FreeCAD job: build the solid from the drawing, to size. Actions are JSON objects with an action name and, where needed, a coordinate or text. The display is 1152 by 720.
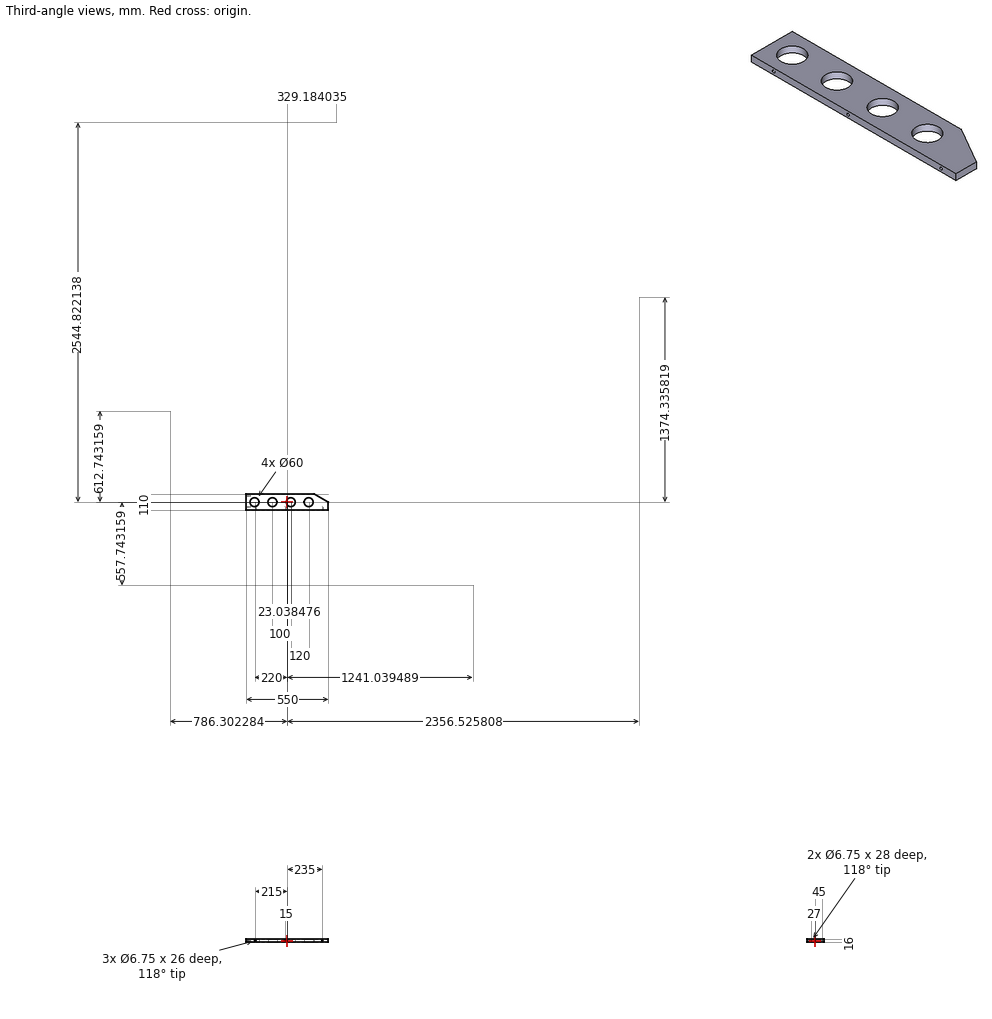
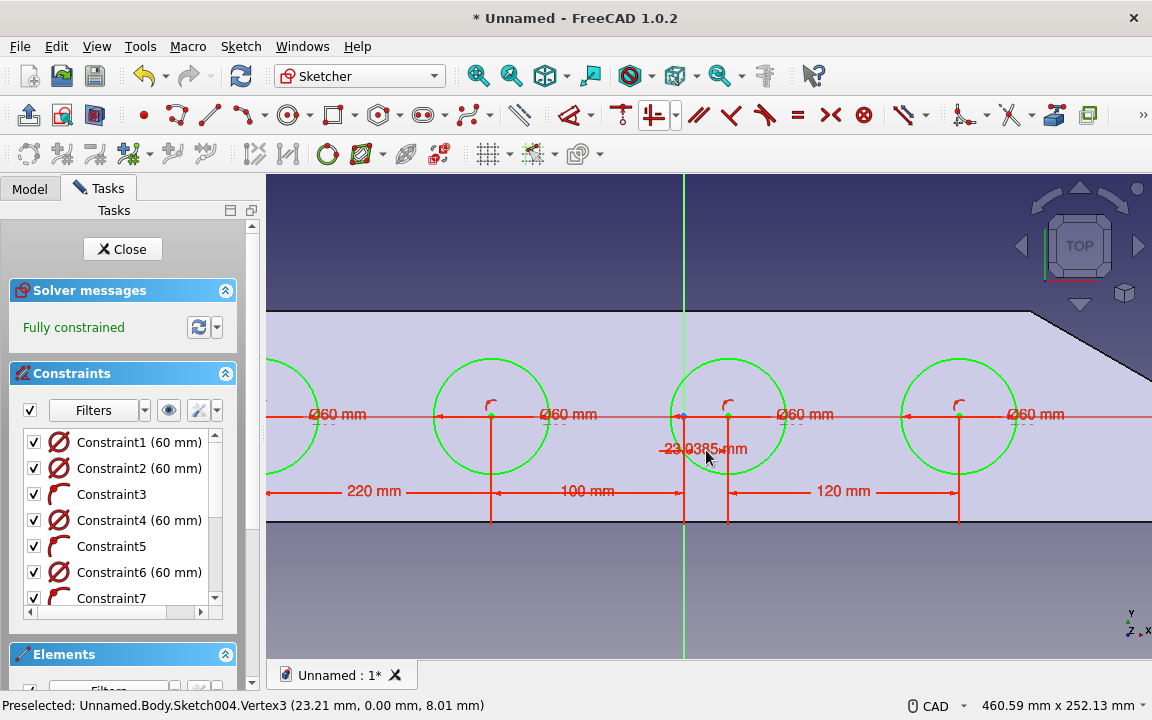
{"action": "left_click", "coordinate": [123, 249]}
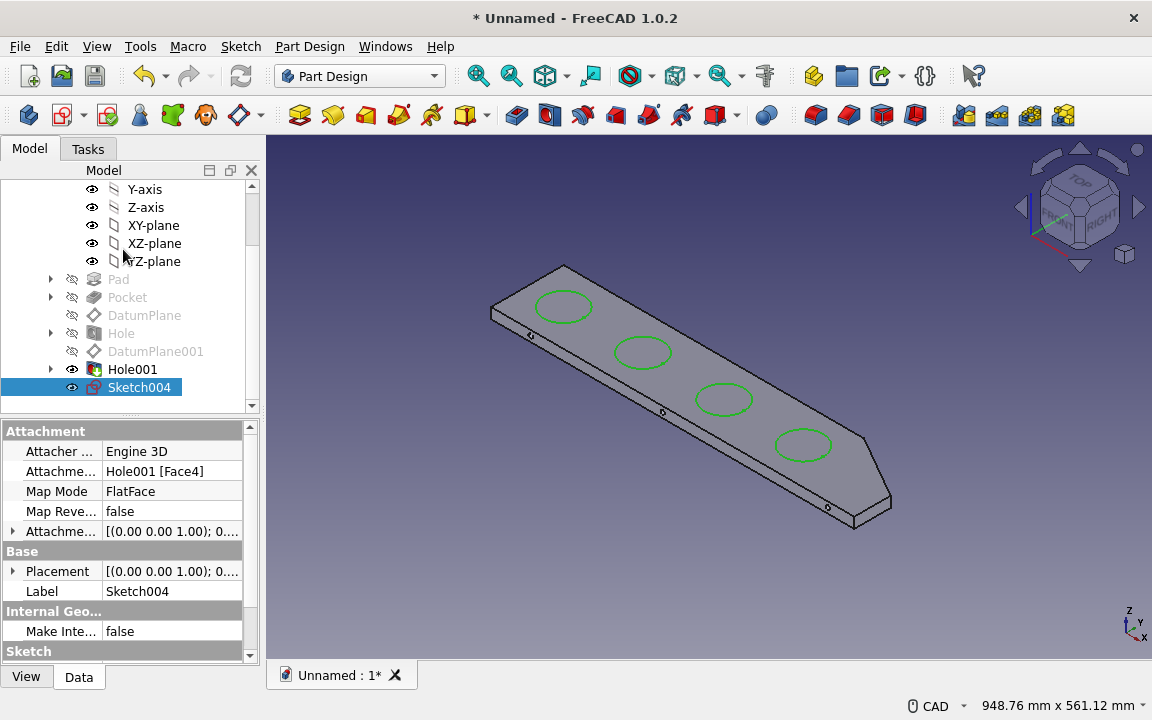
{"action": "left_click", "coordinate": [517, 116]}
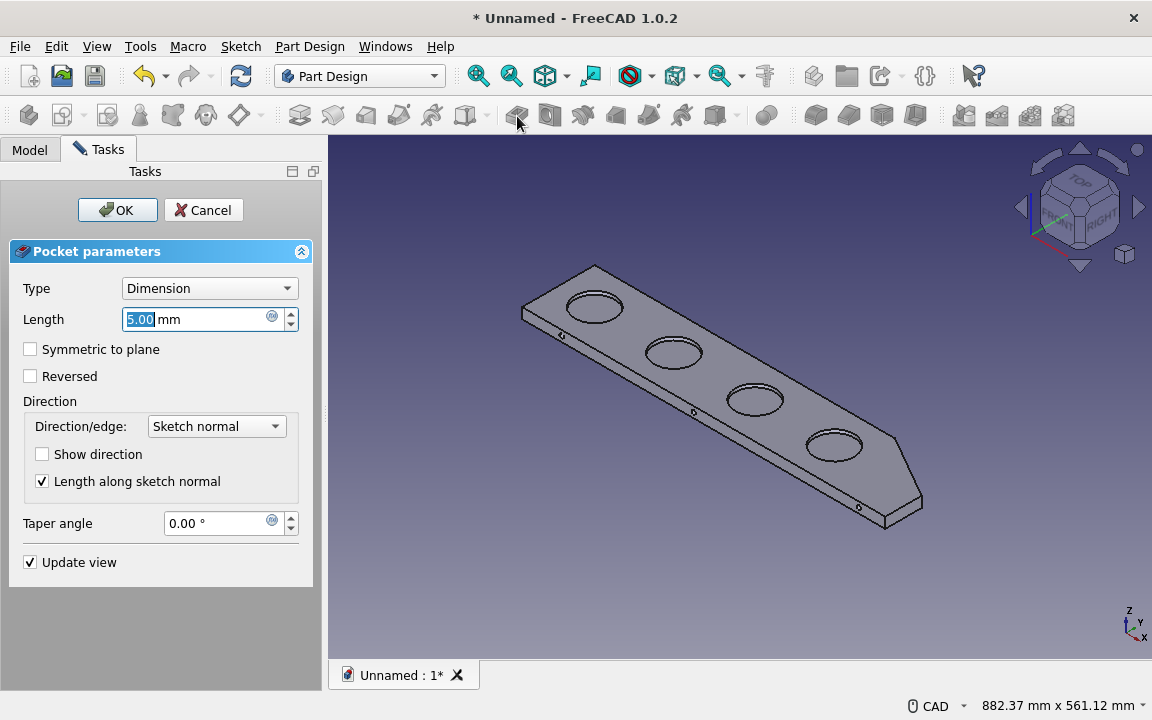
{"action": "left_click", "coordinate": [210, 288]}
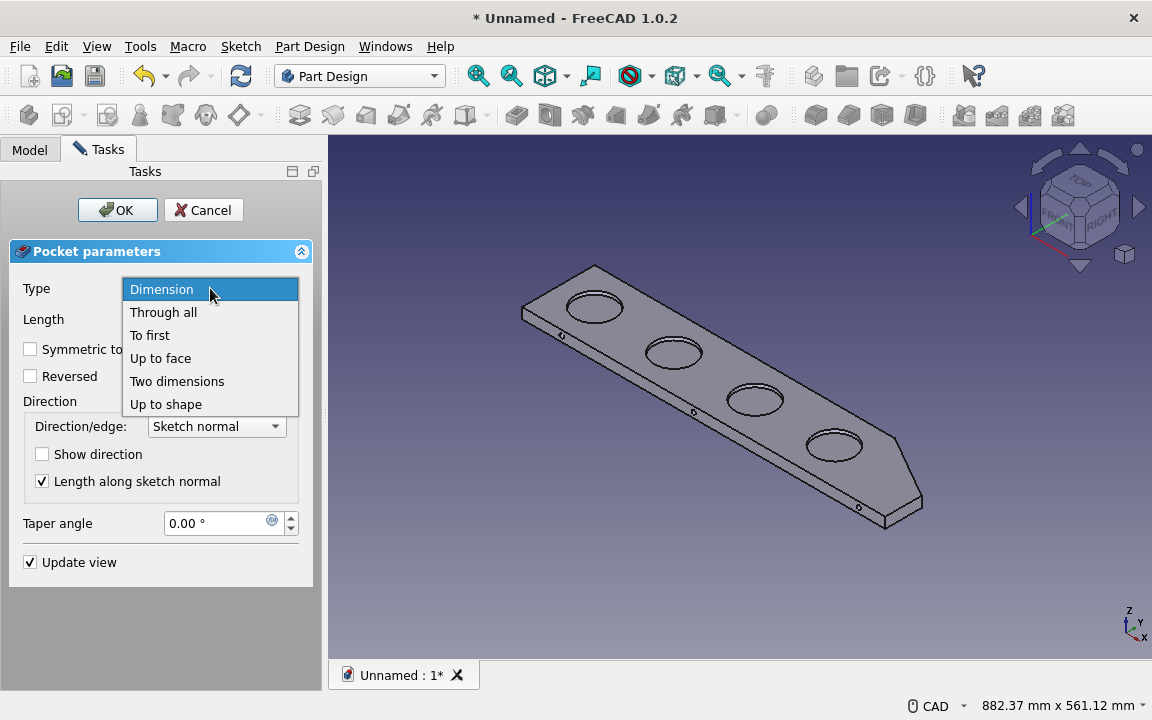
{"action": "left_click", "coordinate": [208, 312]}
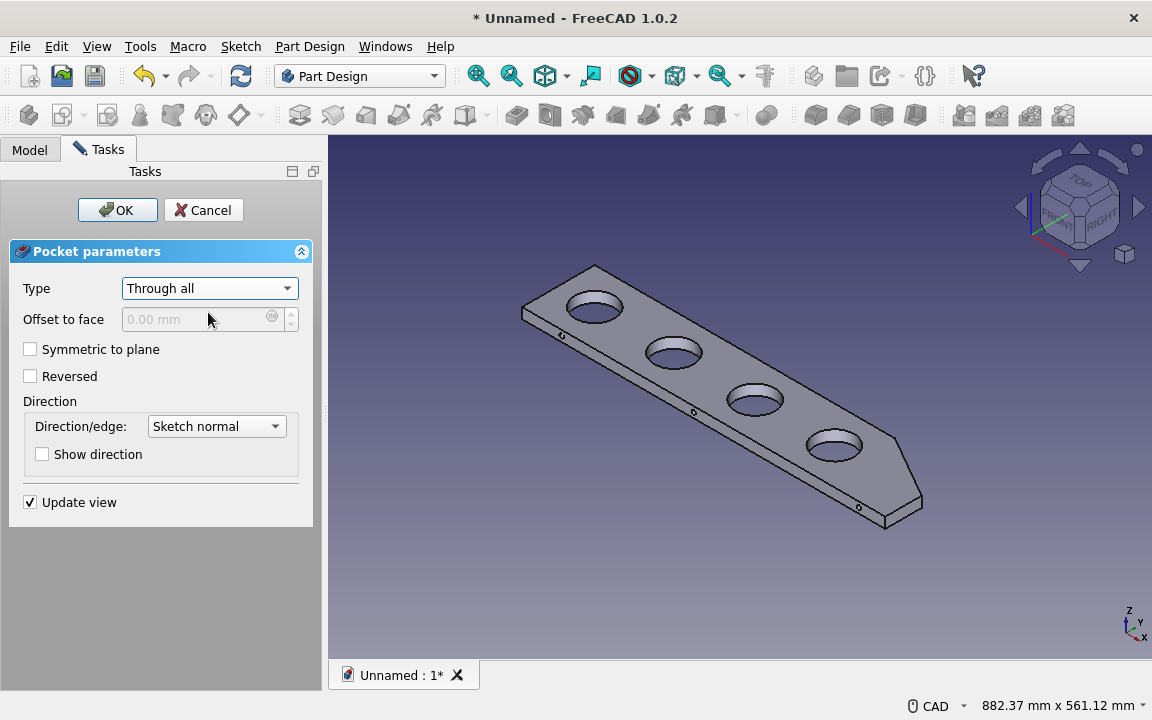
{"action": "left_click", "coordinate": [118, 210]}